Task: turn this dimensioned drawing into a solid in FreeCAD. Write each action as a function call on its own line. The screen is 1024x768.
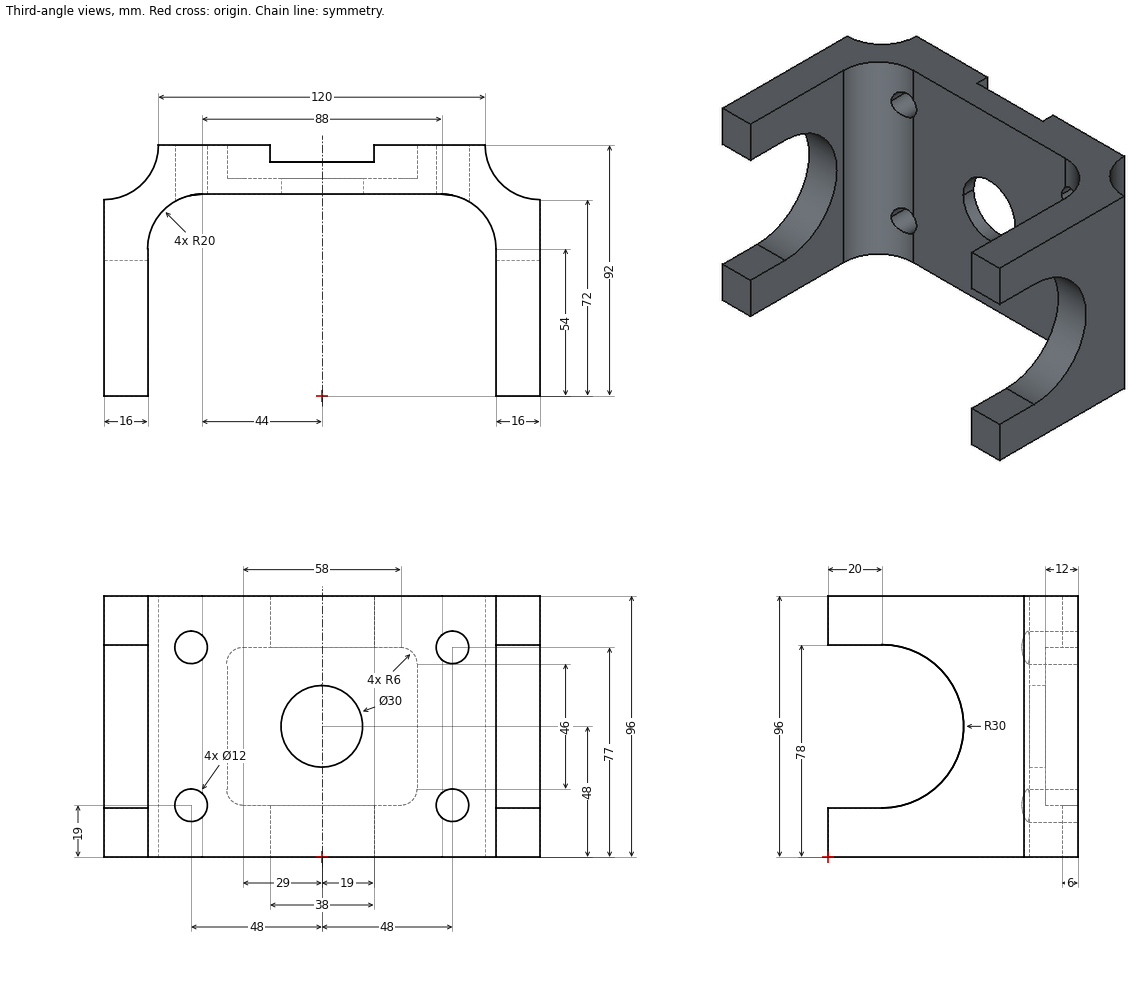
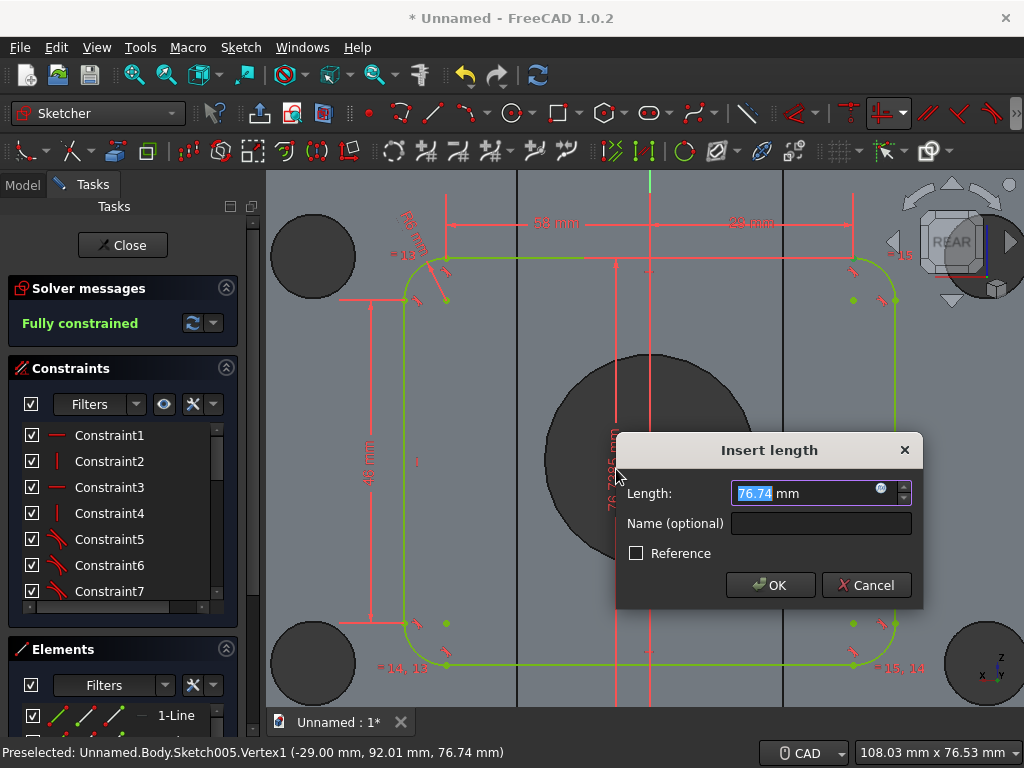
text(77)
key(Return)
key(Escape)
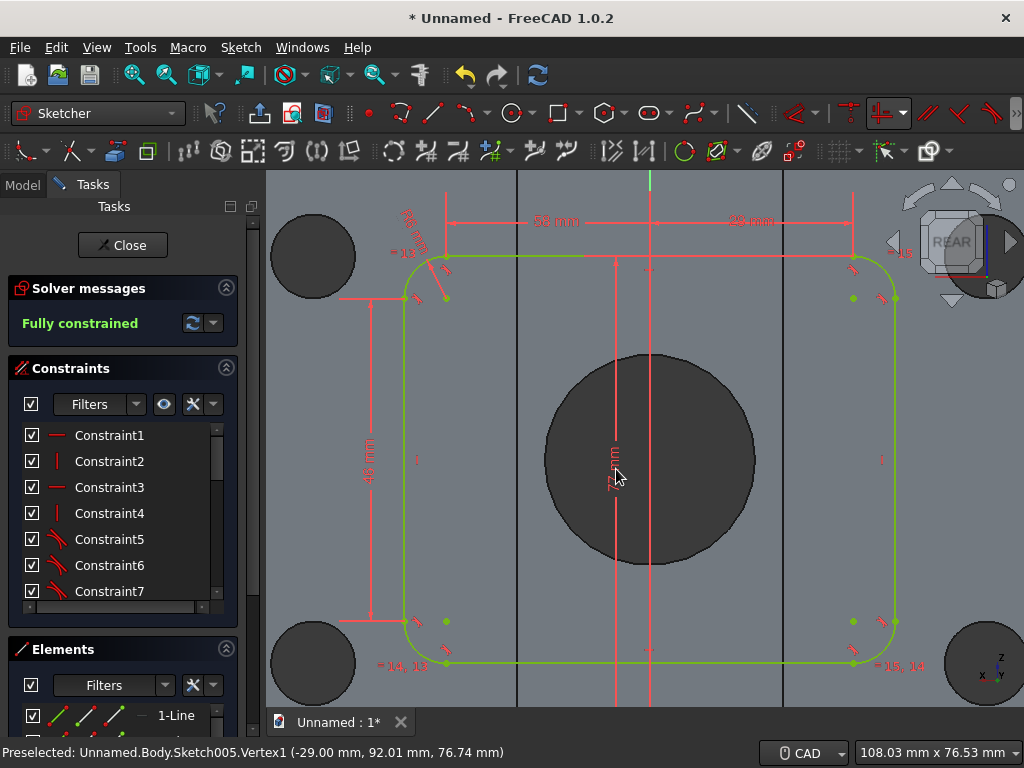
click(123, 245)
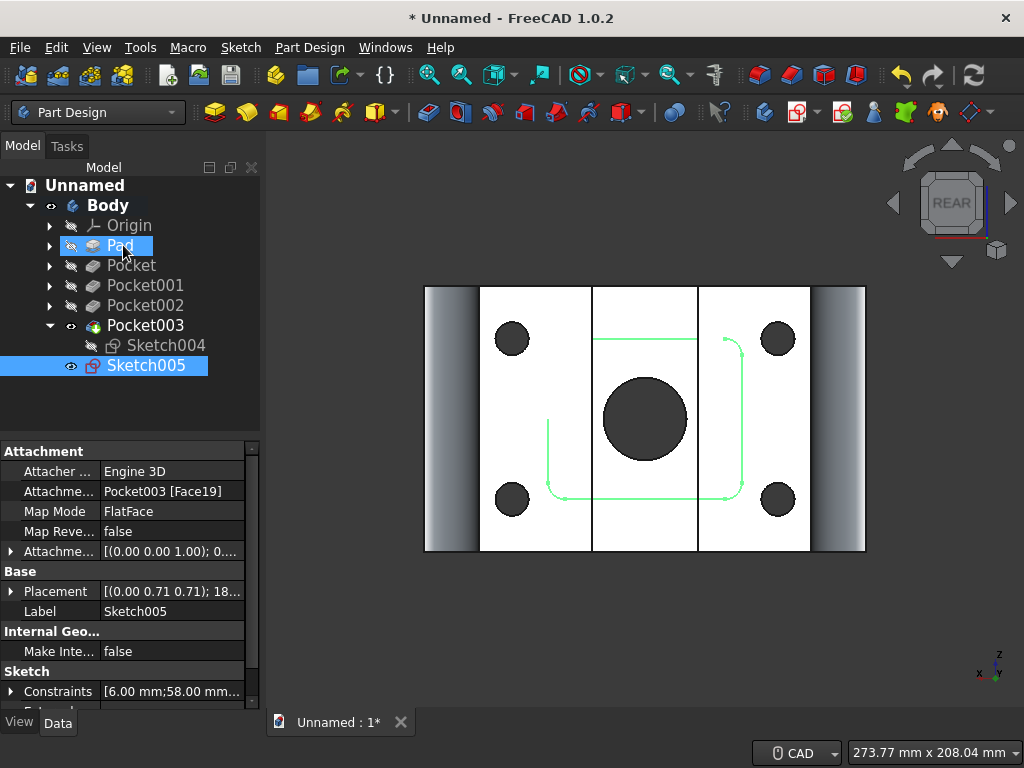
click(430, 112)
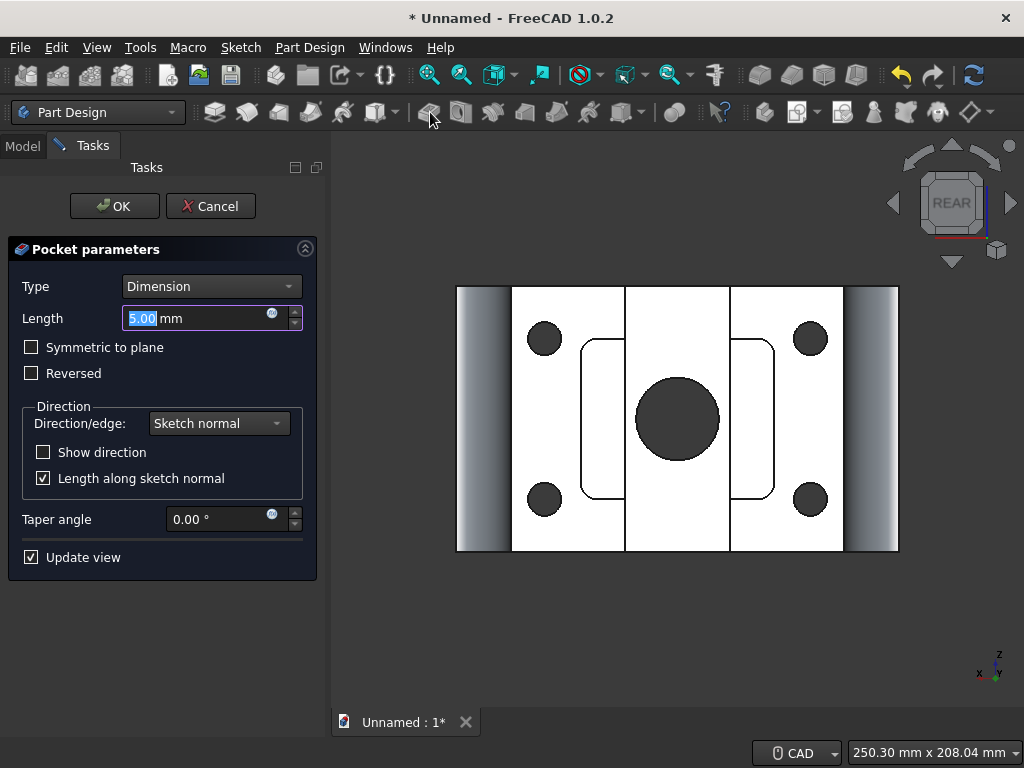
text(12)
key(Tab)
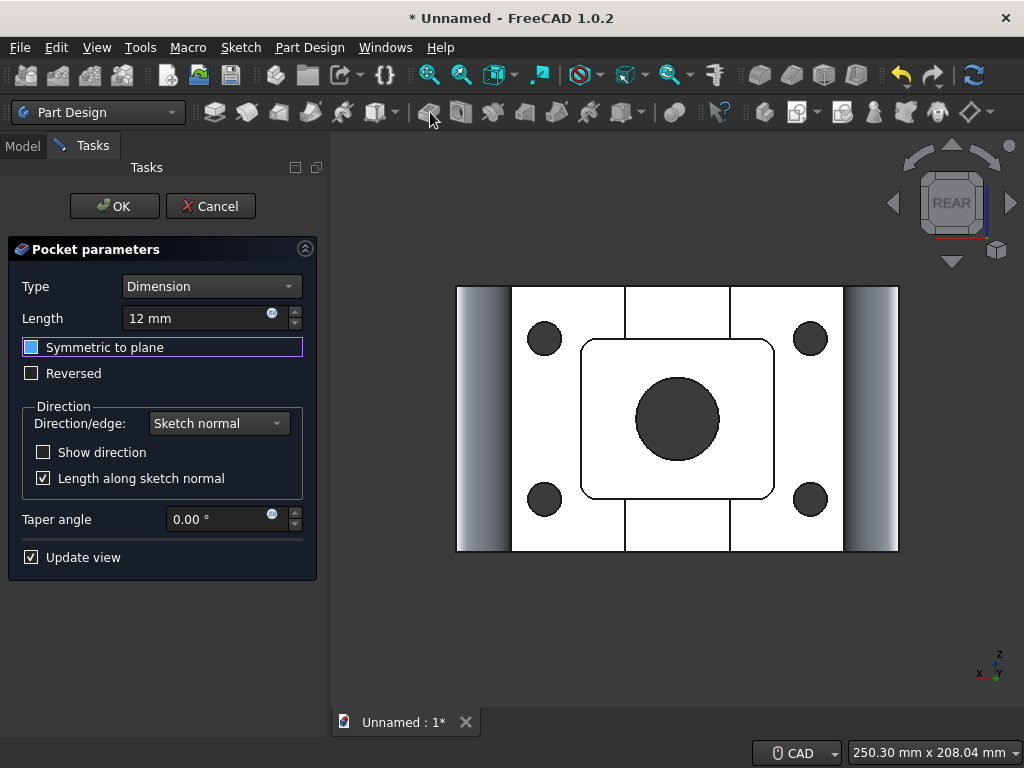
click(115, 206)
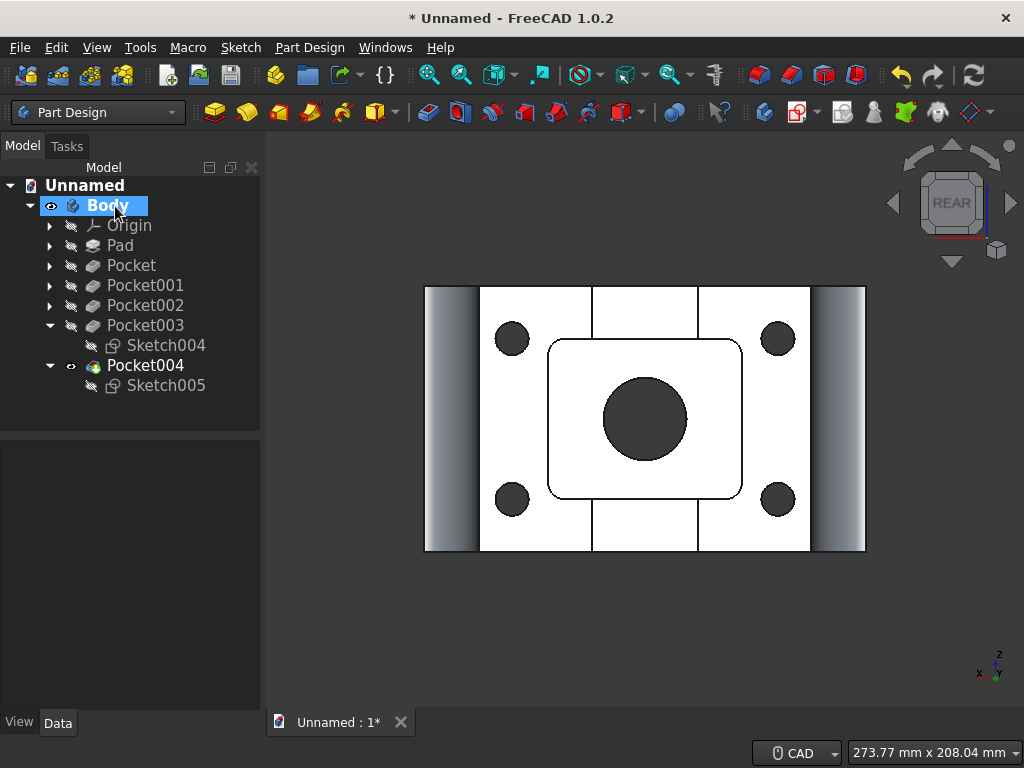
key(0)